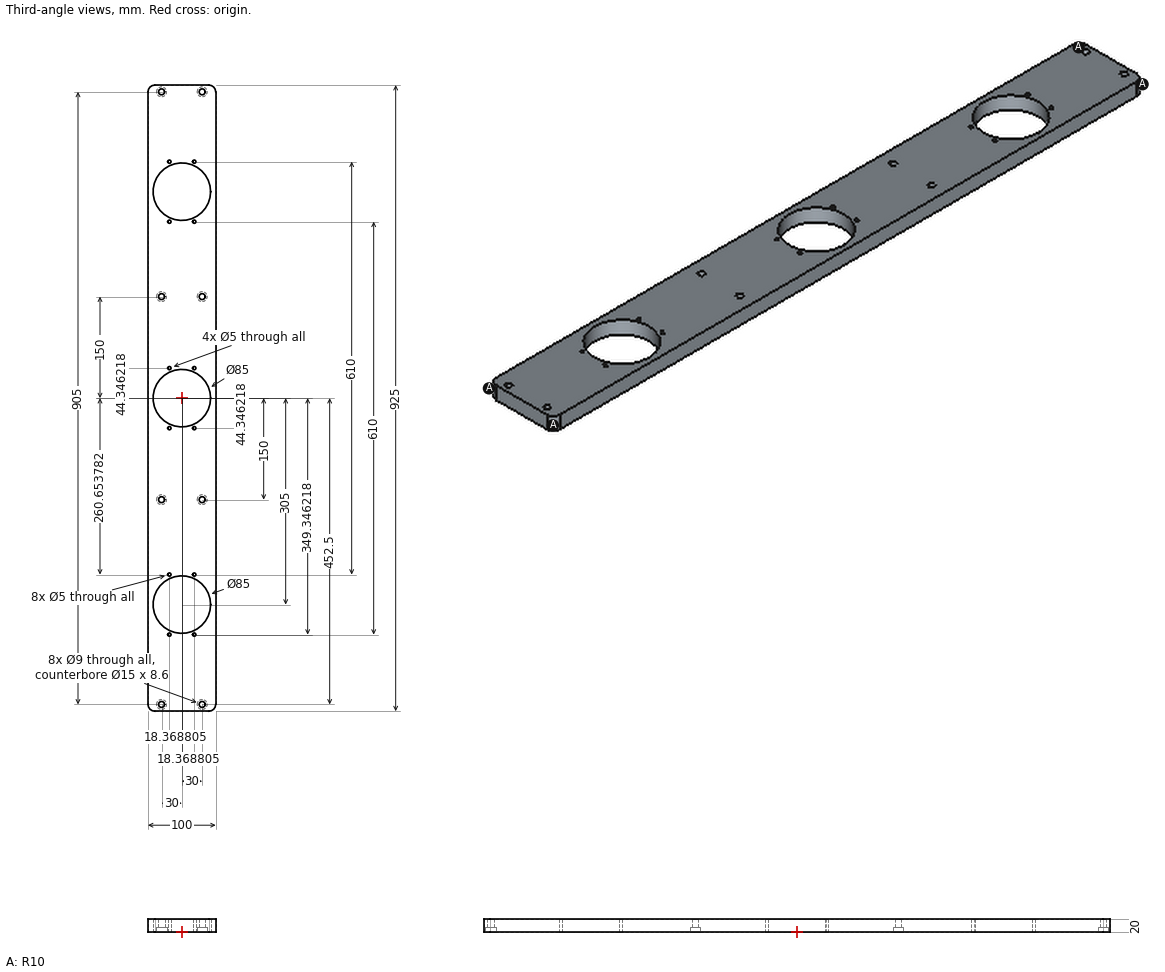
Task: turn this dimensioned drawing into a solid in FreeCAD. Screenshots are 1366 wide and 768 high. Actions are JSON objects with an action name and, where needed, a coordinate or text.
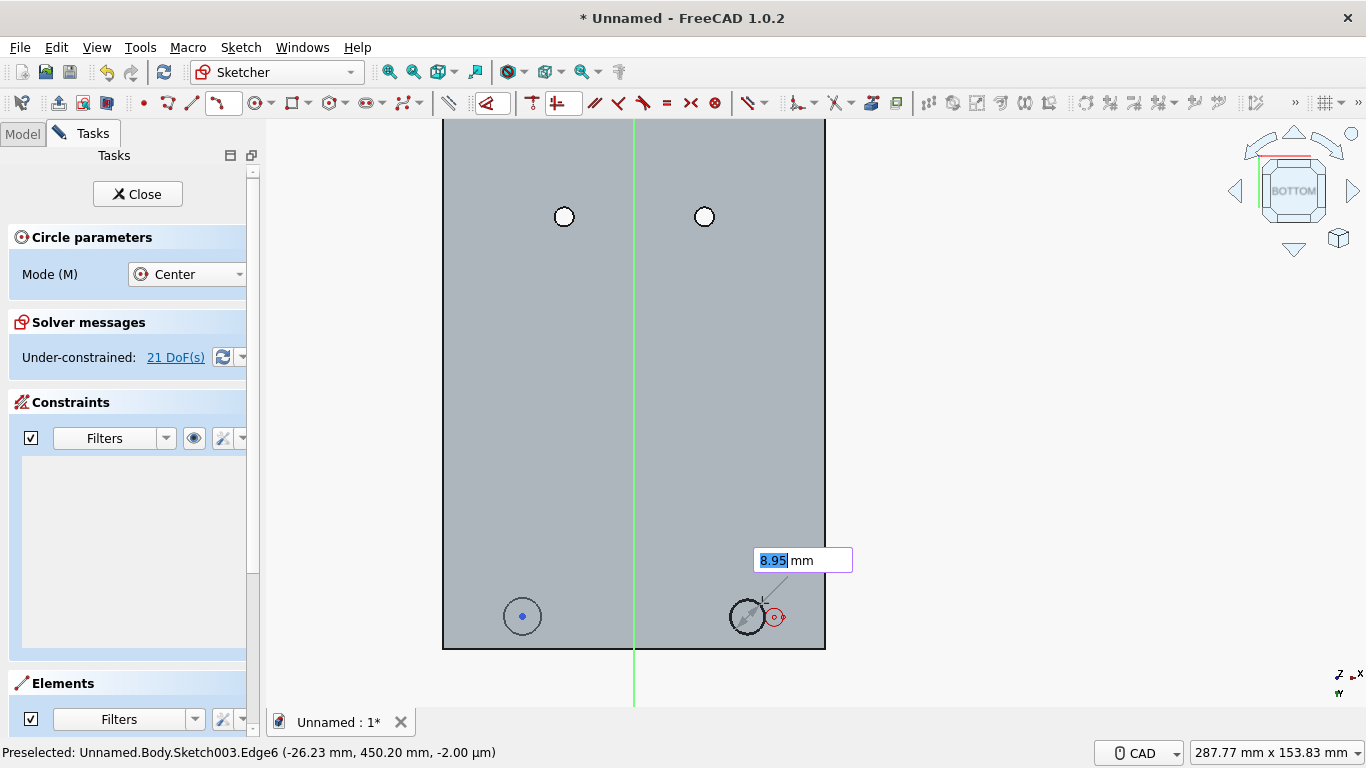
{"action": "left_click", "coordinate": [761, 599]}
{"action": "key", "text": "Escape"}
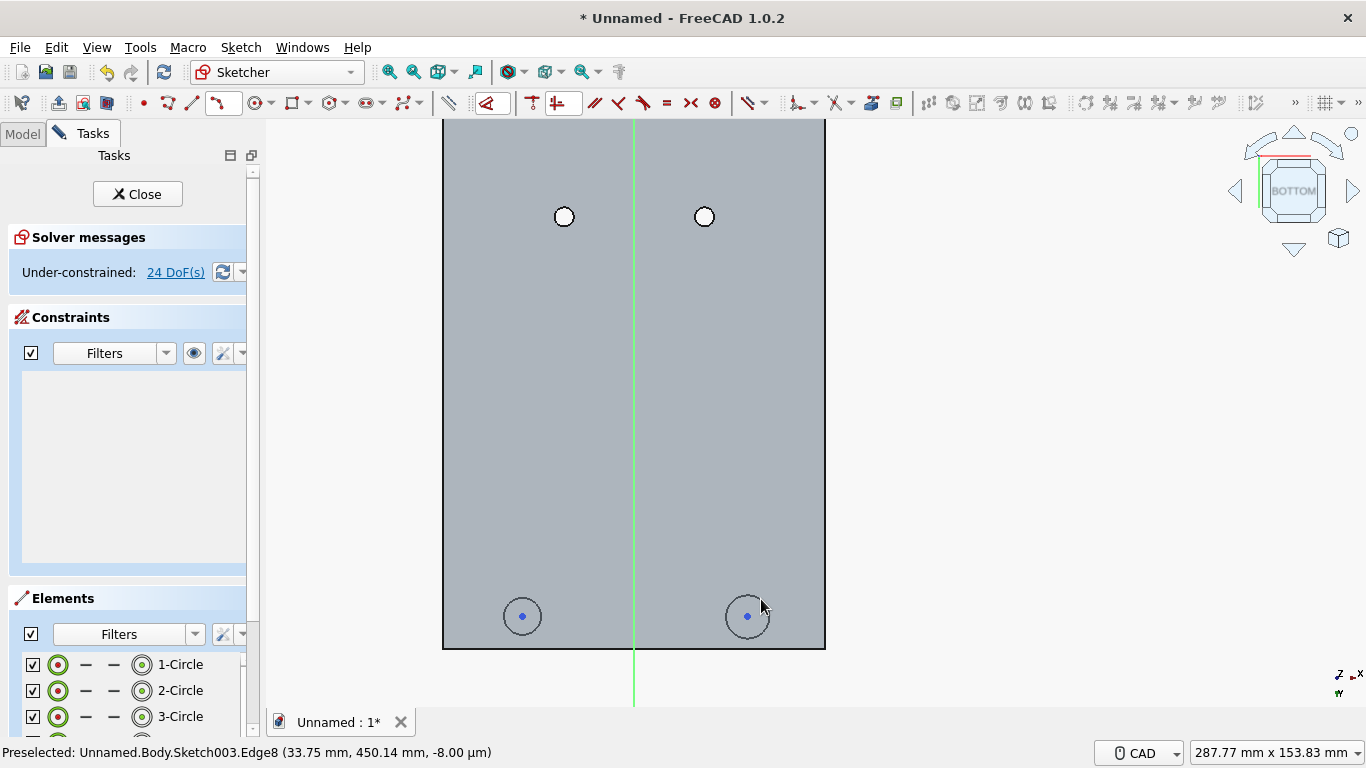
{"action": "scroll", "coordinate": [762, 604], "scroll_direction": "down", "scroll_amount": 11}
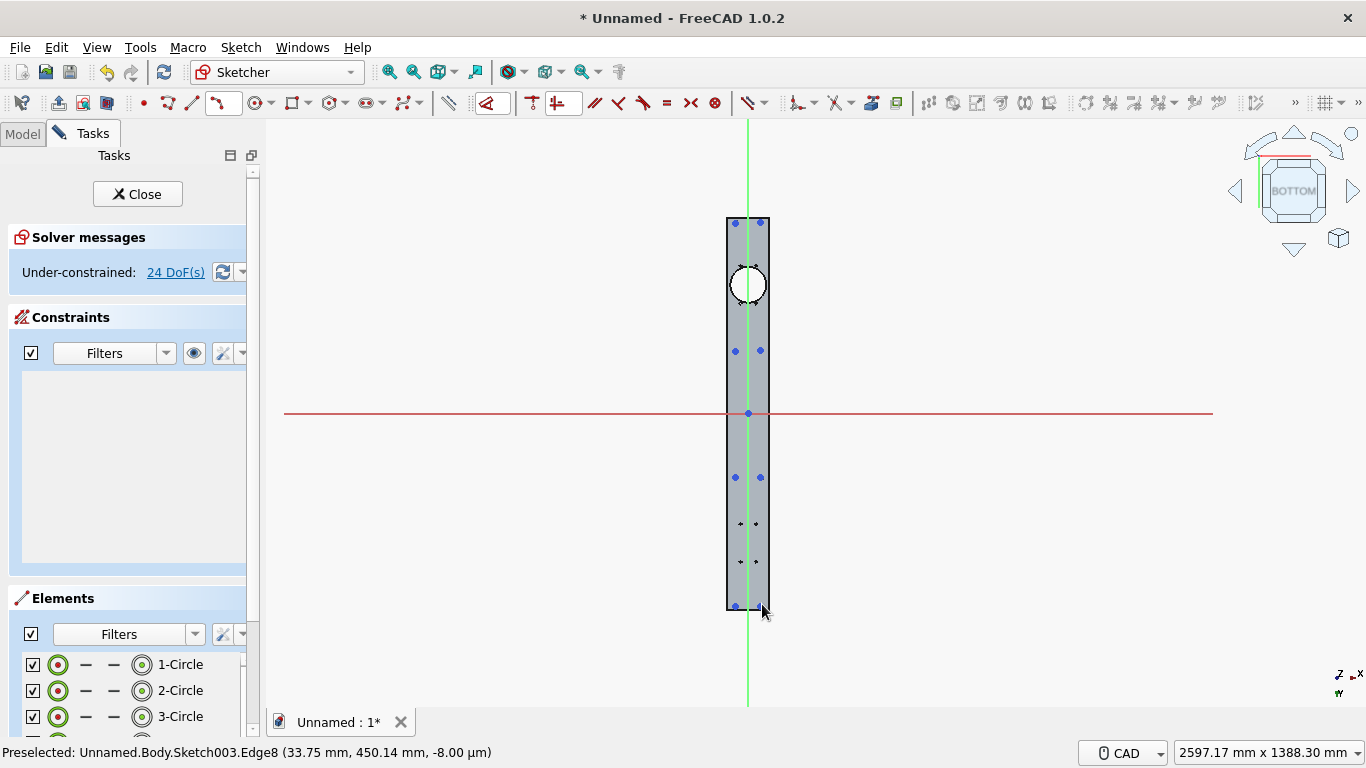
{"action": "scroll", "coordinate": [763, 221], "scroll_direction": "up", "scroll_amount": 9}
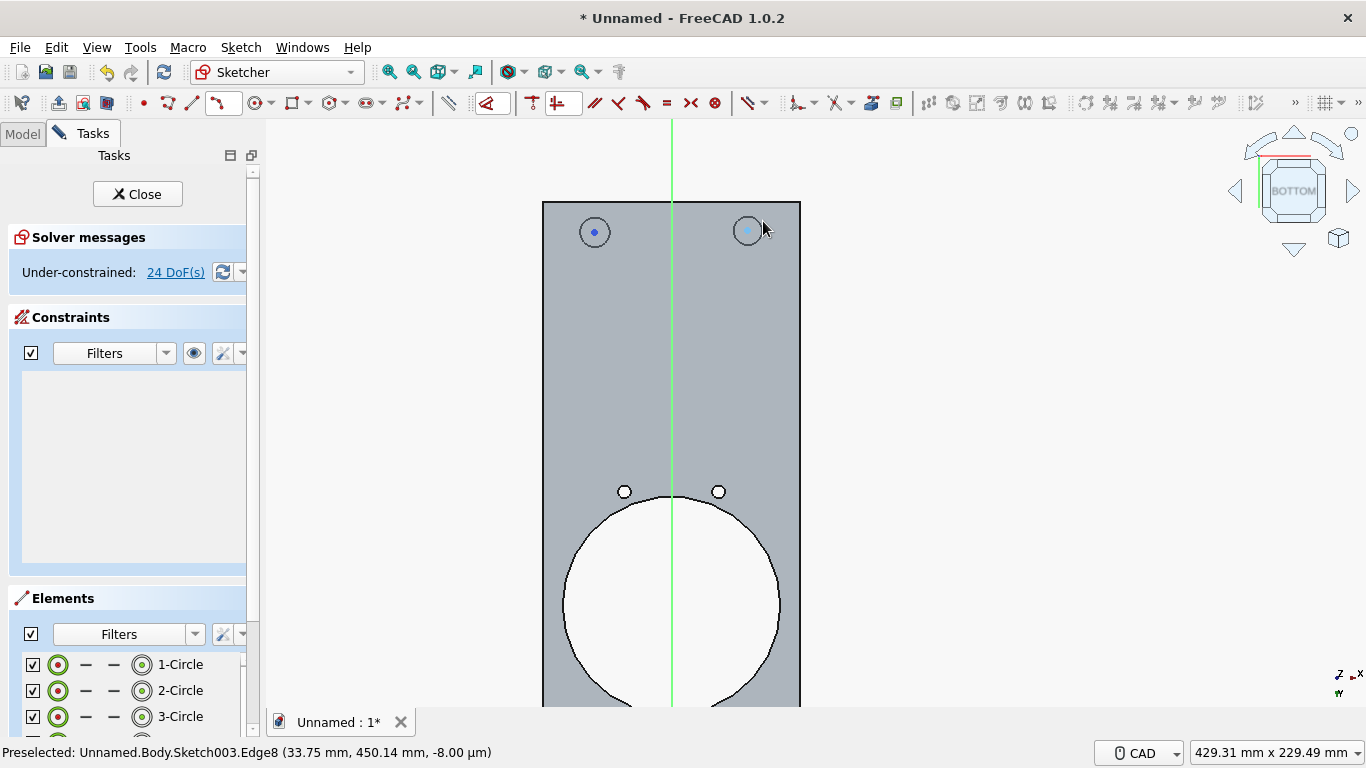
{"action": "left_click", "coordinate": [758, 221]}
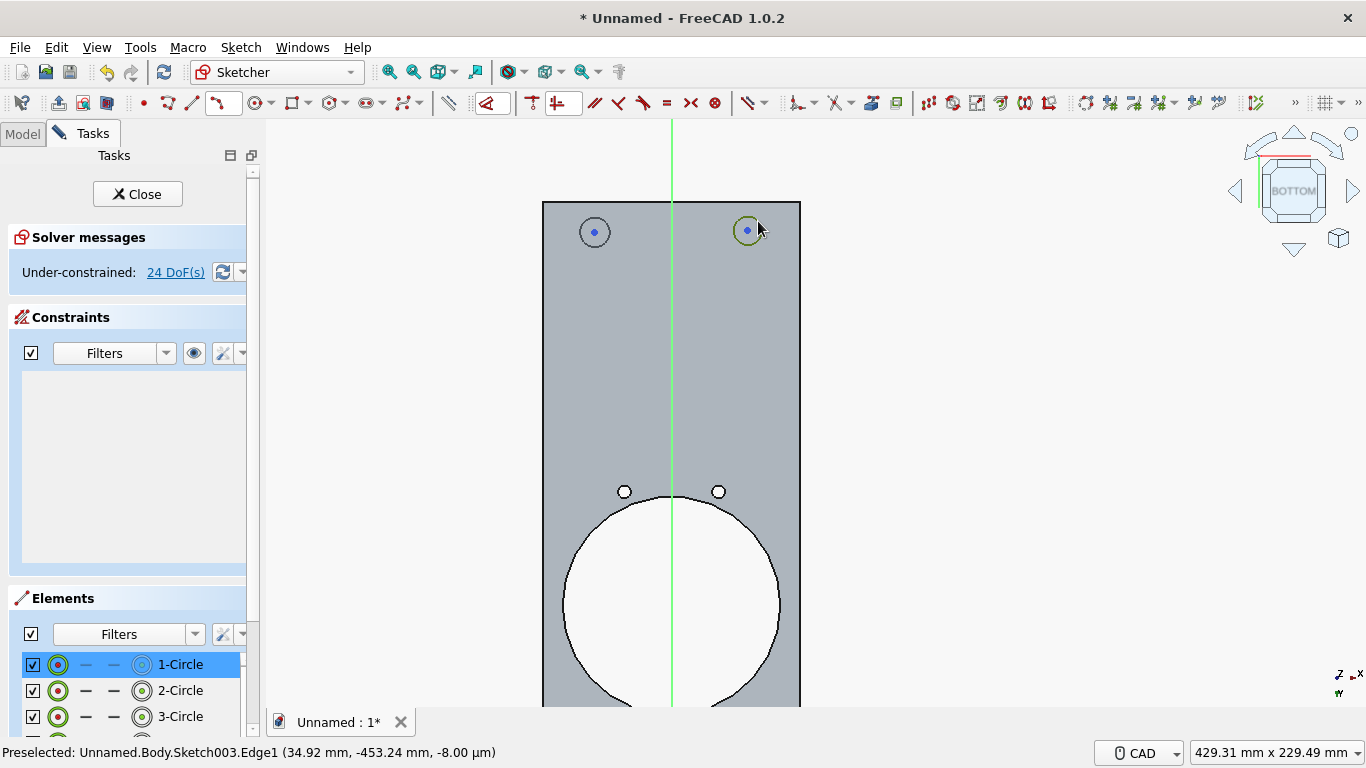
{"action": "left_click", "coordinate": [605, 222]}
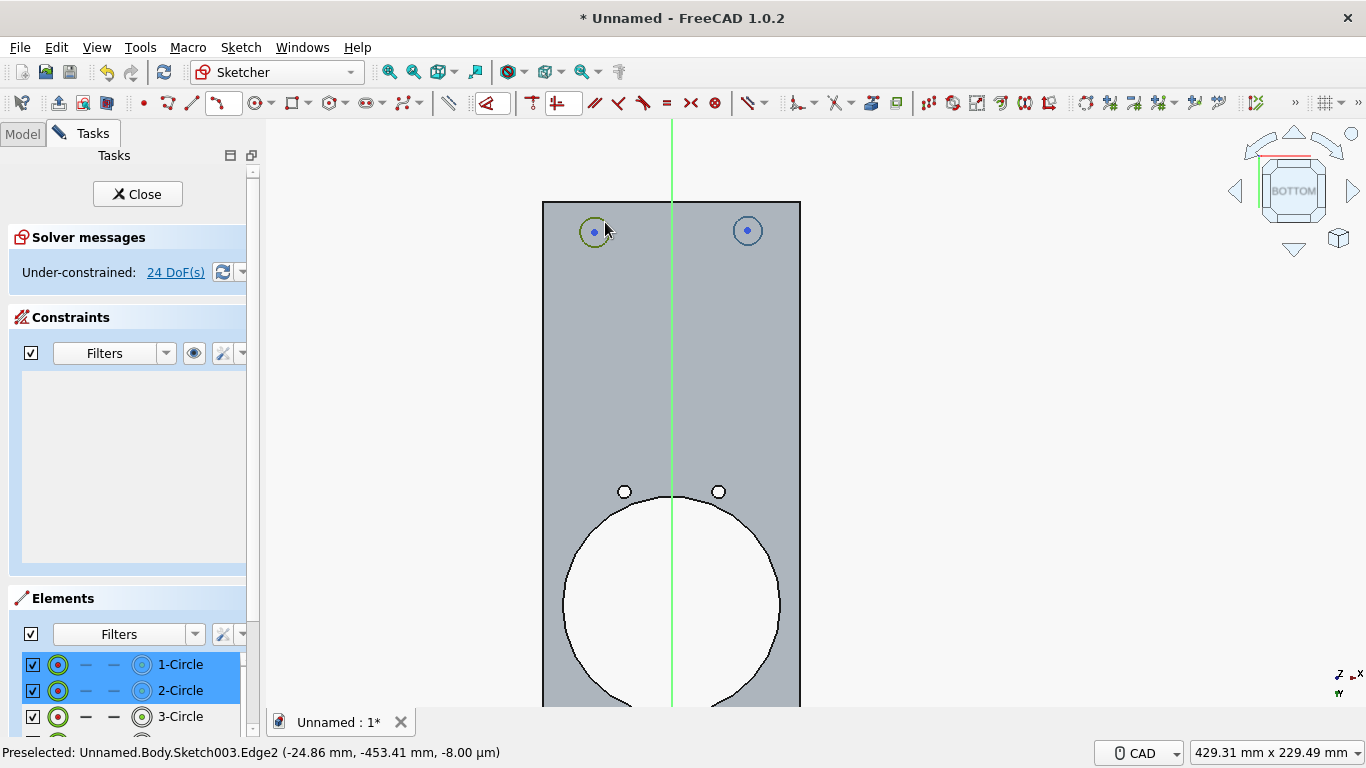
{"action": "scroll", "coordinate": [763, 220], "scroll_direction": "down", "scroll_amount": 9}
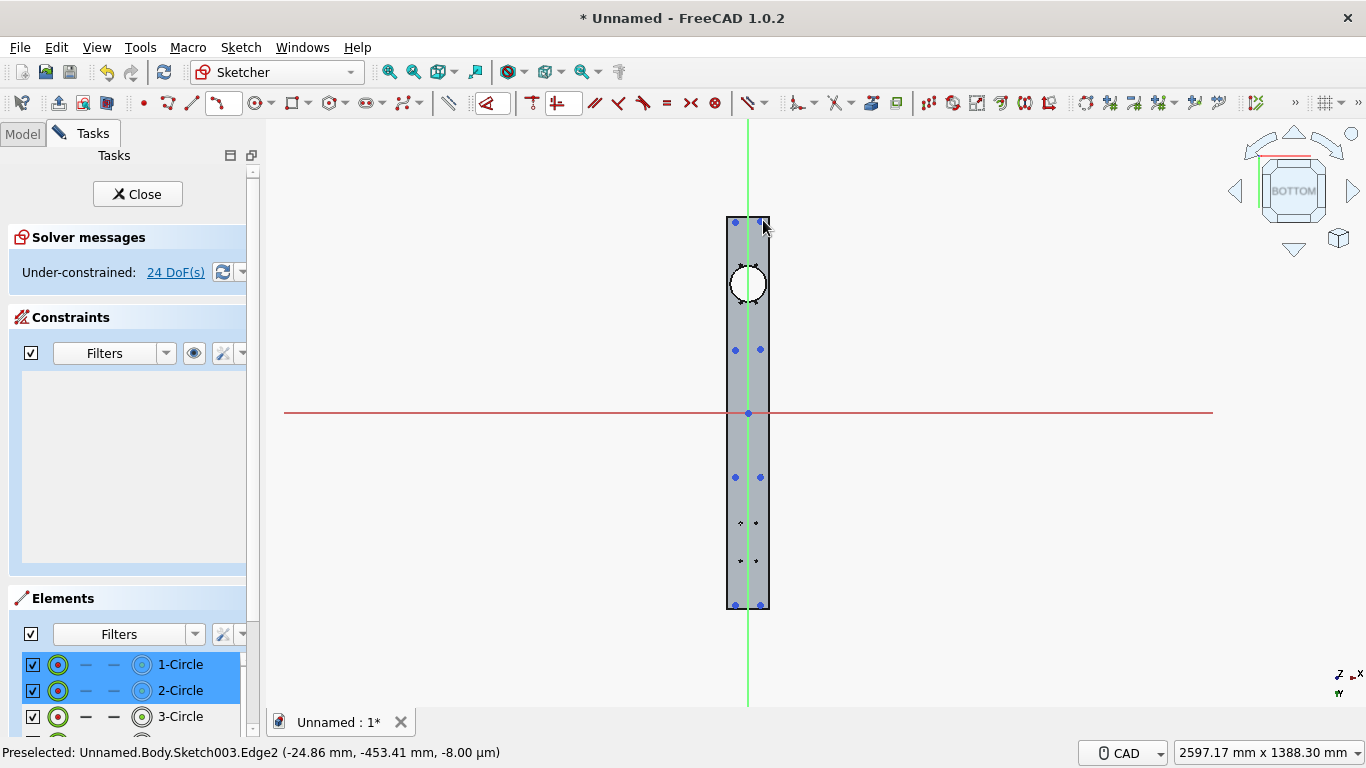
{"action": "scroll", "coordinate": [762, 348], "scroll_direction": "up", "scroll_amount": 10}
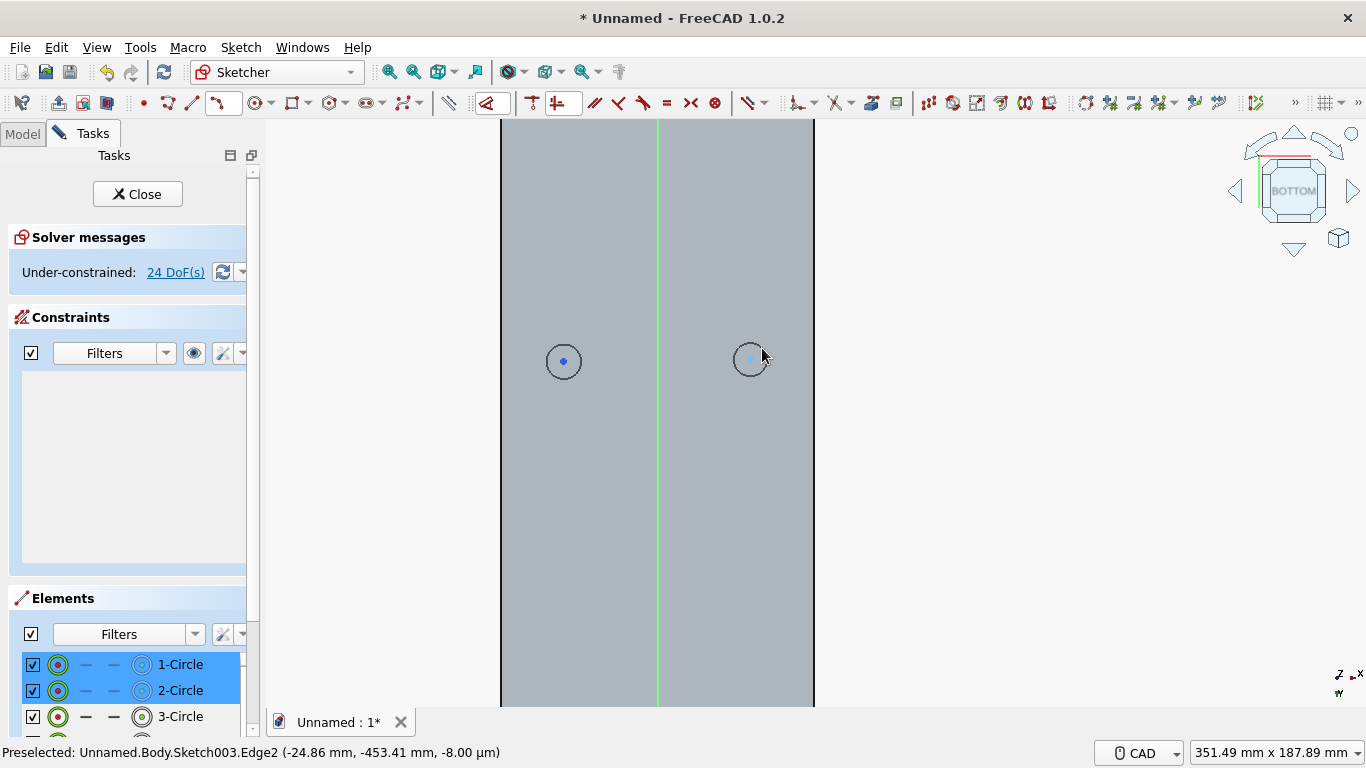
{"action": "left_click", "coordinate": [762, 348]}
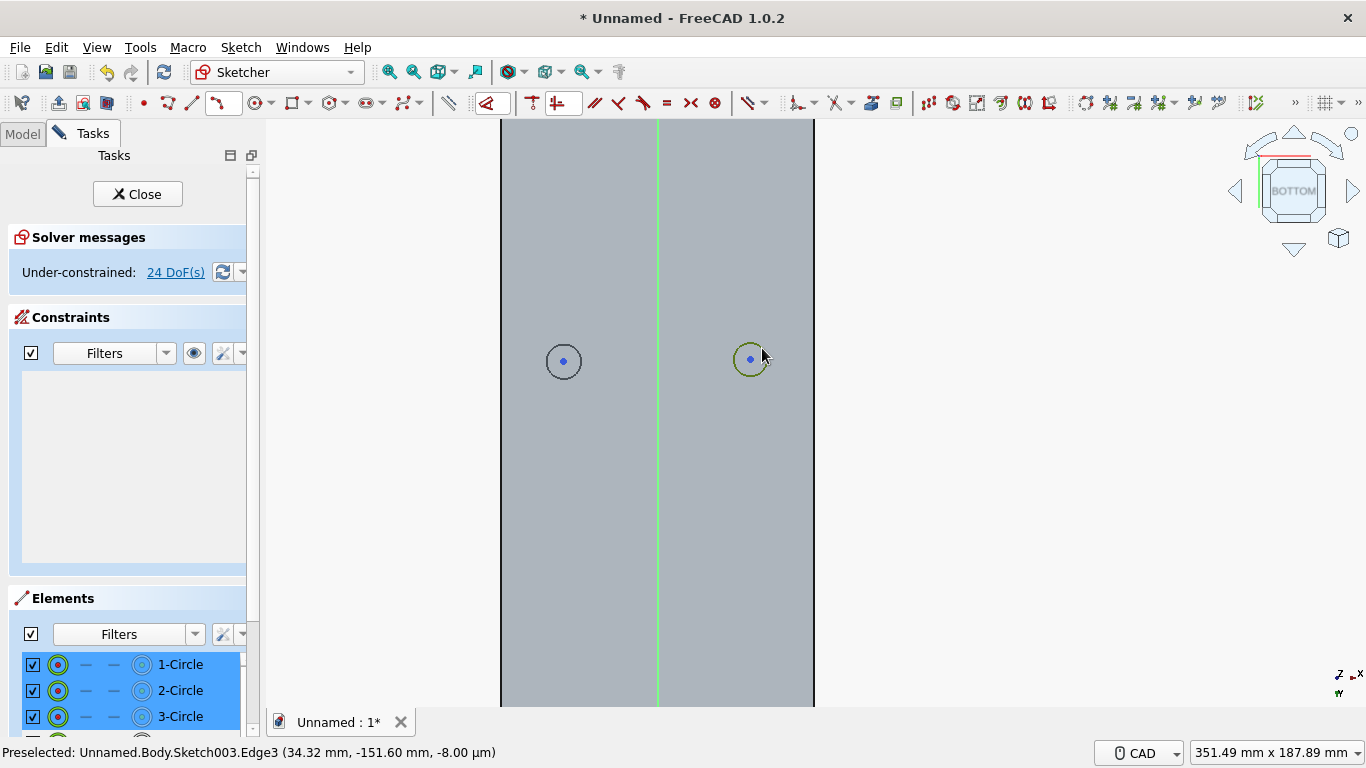
{"action": "left_click", "coordinate": [576, 350]}